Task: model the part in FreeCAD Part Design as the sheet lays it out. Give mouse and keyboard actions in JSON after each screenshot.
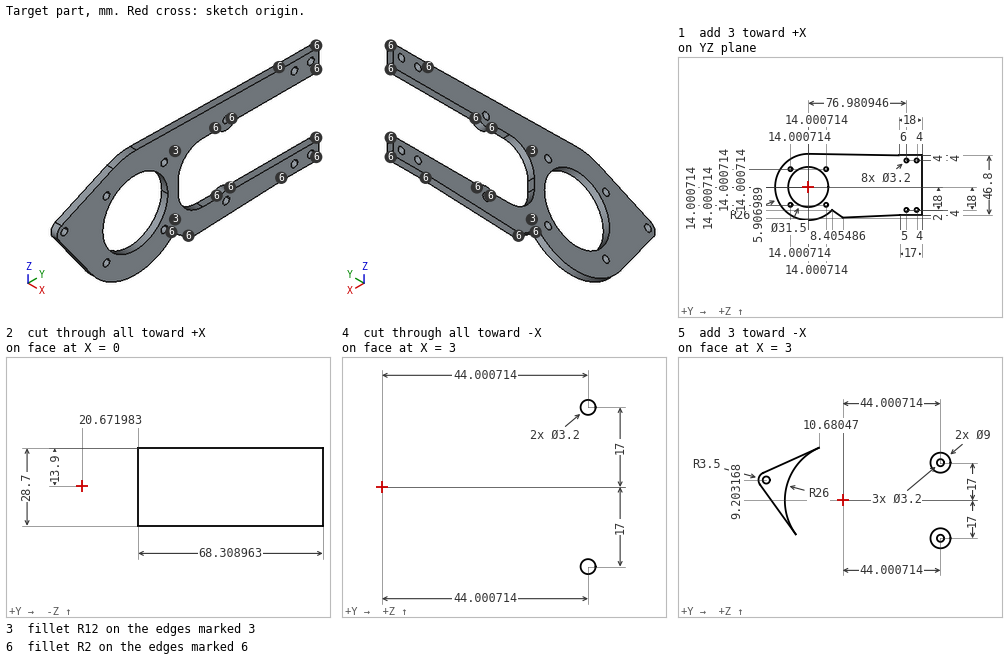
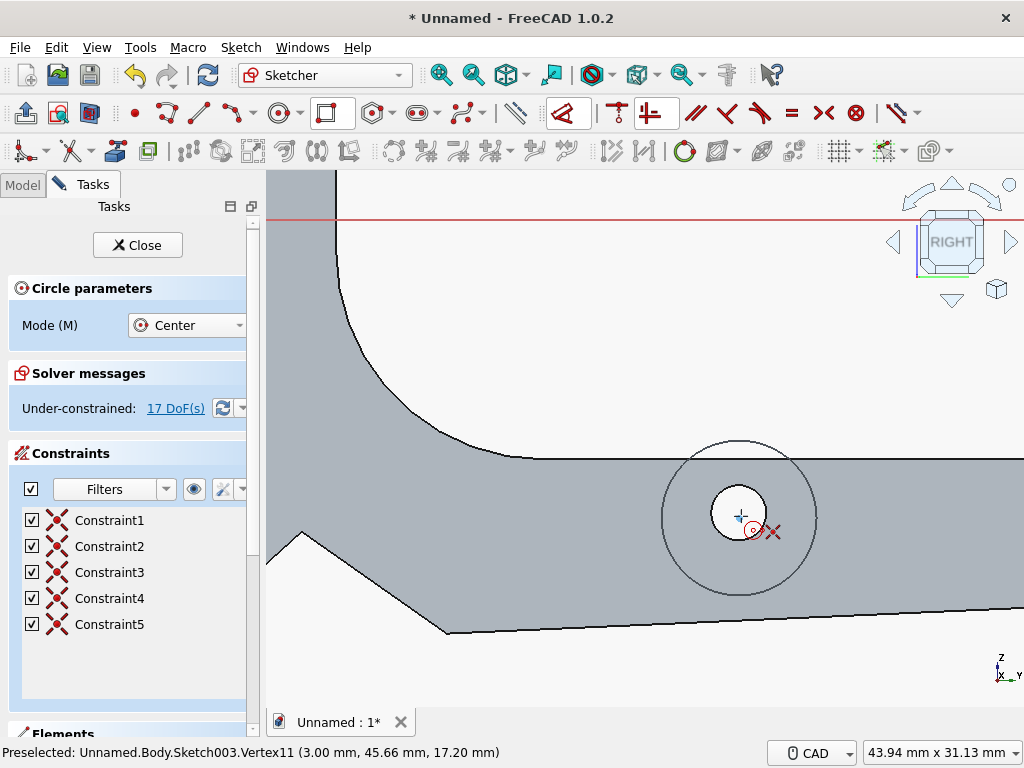
{"action": "scroll", "coordinate": [741, 516], "scroll_direction": "down", "scroll_amount": 7}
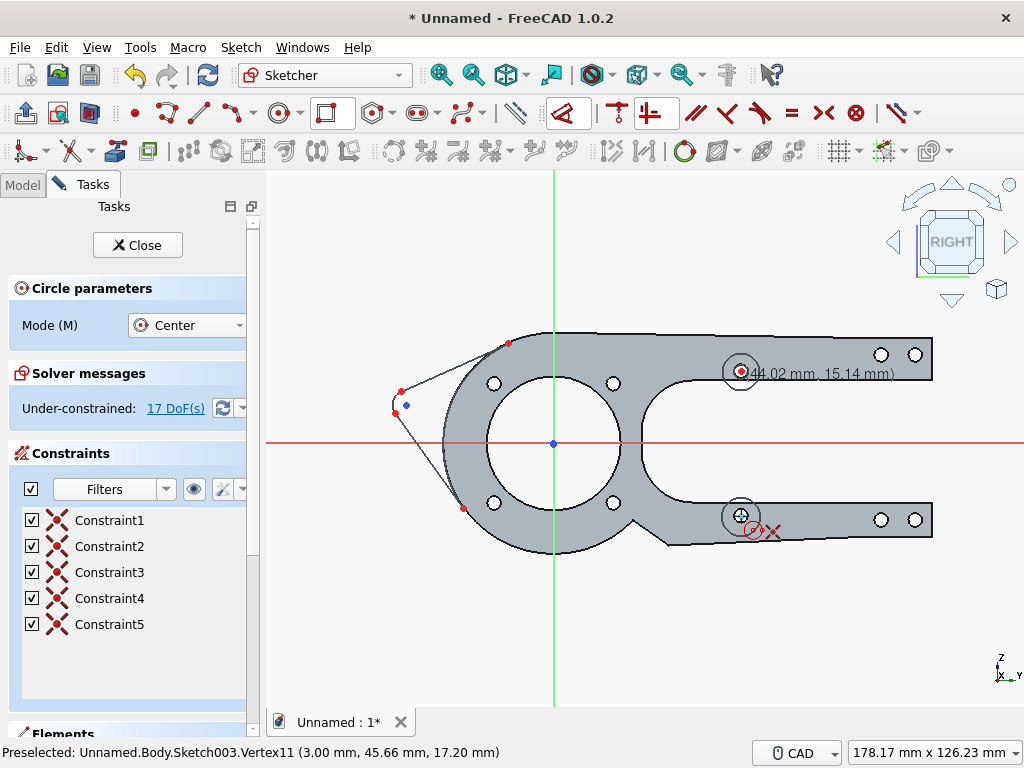
{"action": "left_click", "coordinate": [741, 517]}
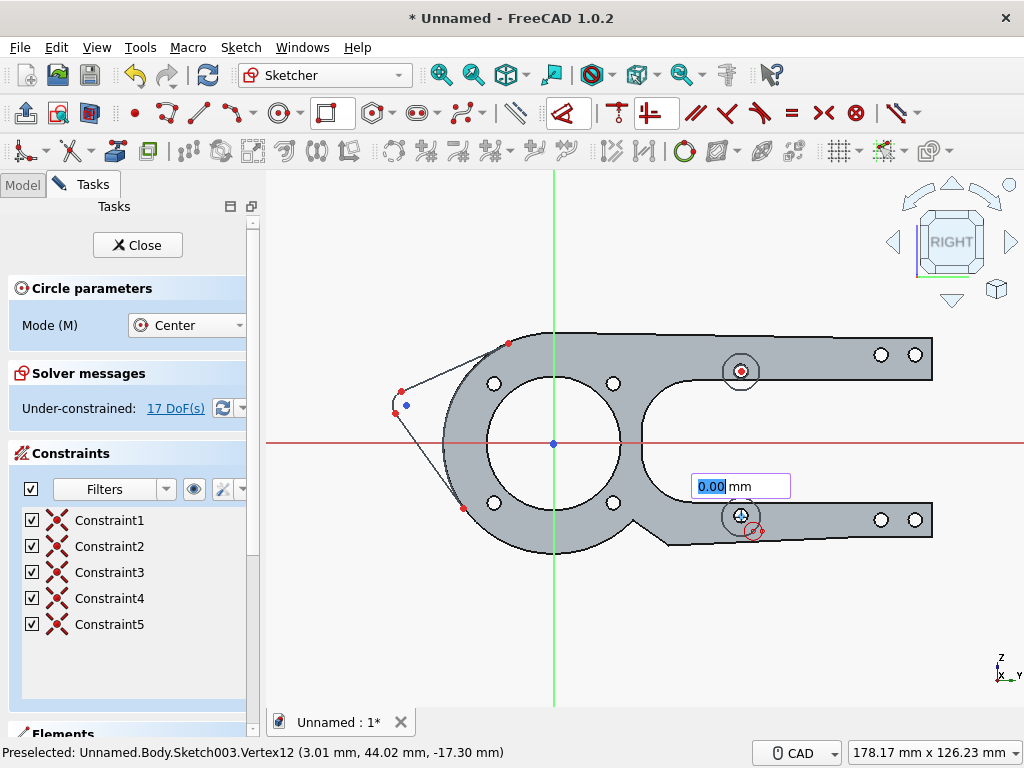
{"action": "scroll", "coordinate": [747, 513], "scroll_direction": "up", "scroll_amount": 5}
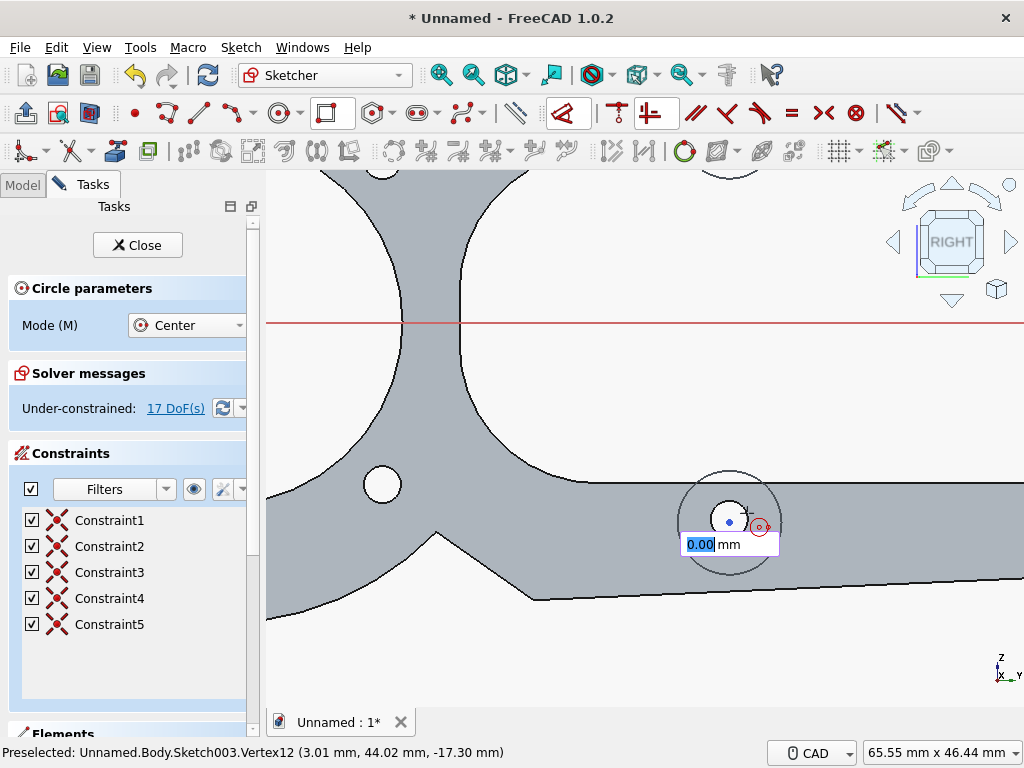
{"action": "left_click", "coordinate": [747, 513]}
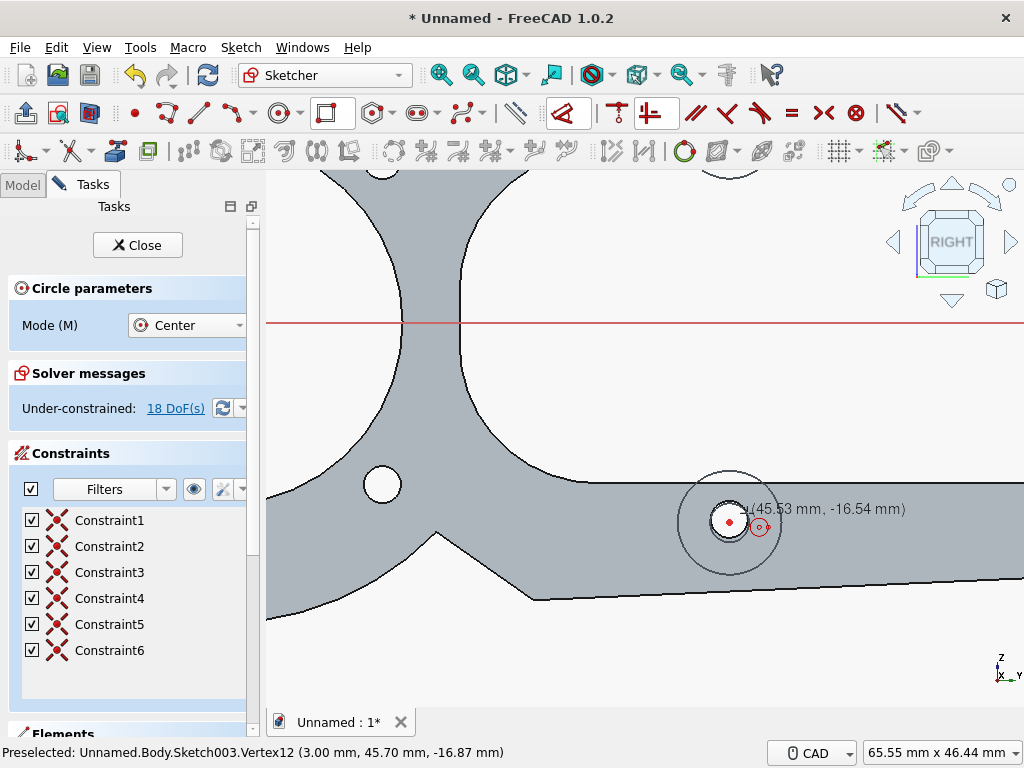
{"action": "scroll", "coordinate": [747, 513], "scroll_direction": "down", "scroll_amount": 5}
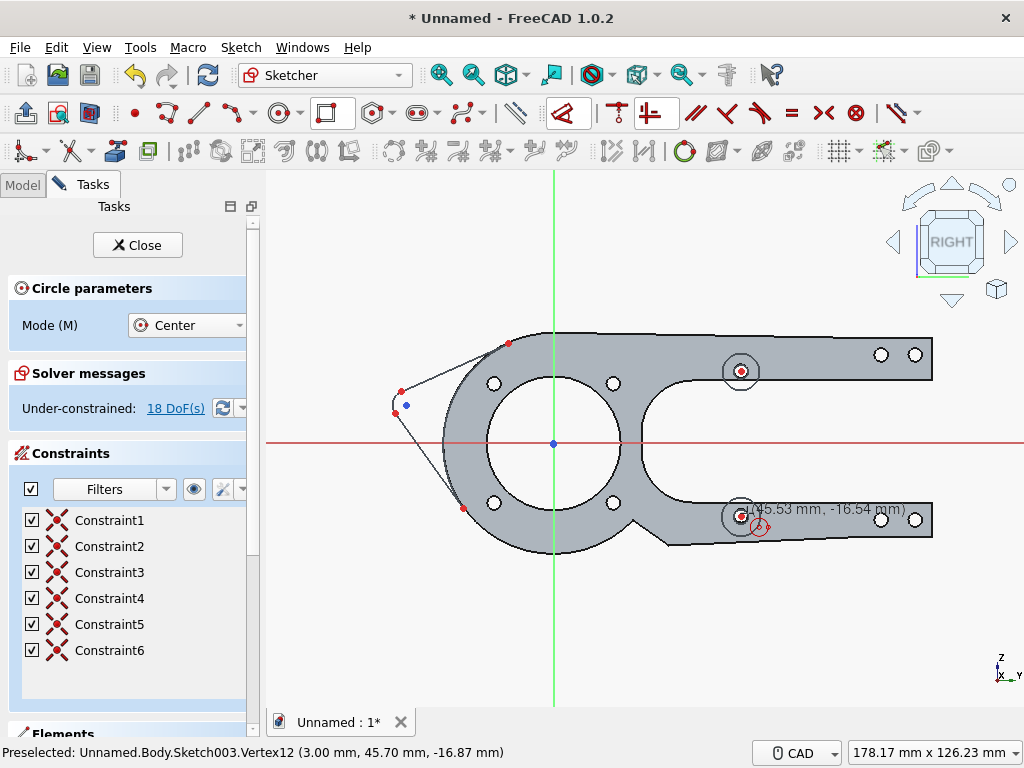
{"action": "scroll", "coordinate": [408, 404], "scroll_direction": "up", "scroll_amount": 7}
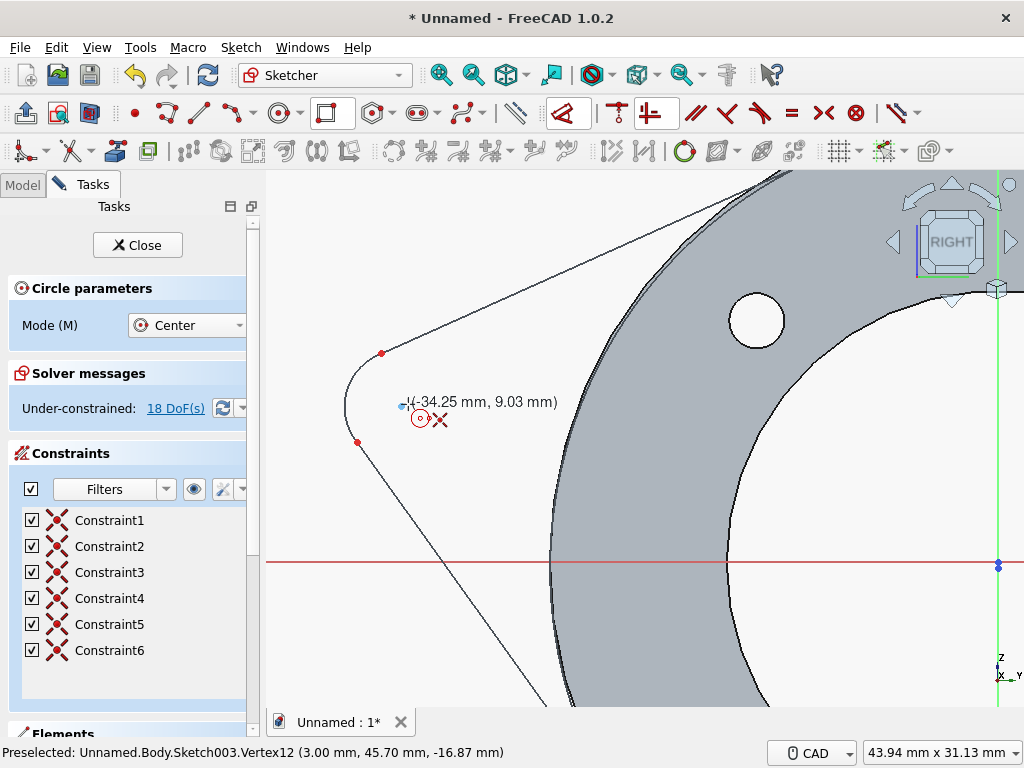
{"action": "scroll", "coordinate": [408, 404], "scroll_direction": "down", "scroll_amount": 7}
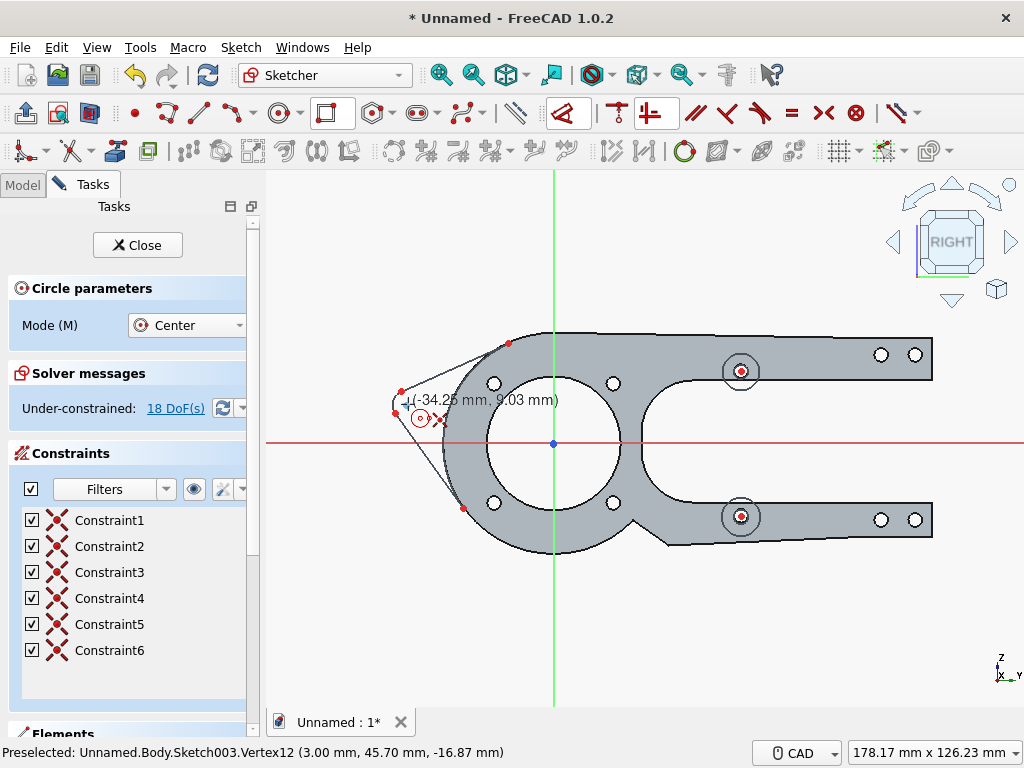
{"action": "left_click", "coordinate": [408, 404]}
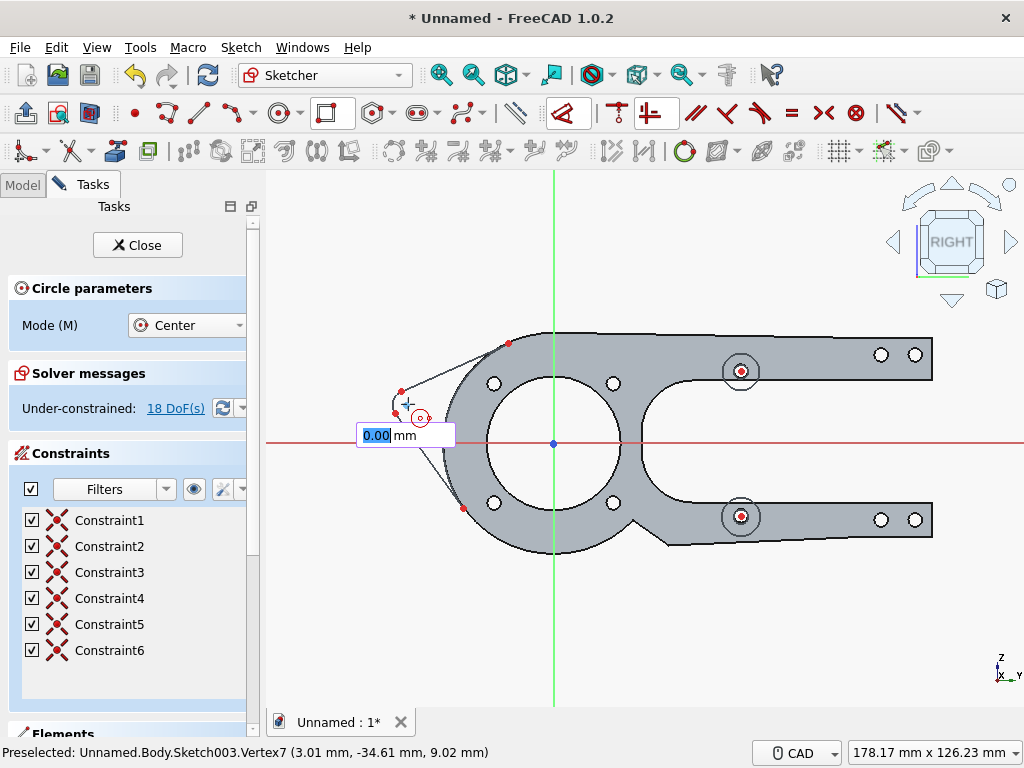
{"action": "scroll", "coordinate": [405, 411], "scroll_direction": "up", "scroll_amount": 5}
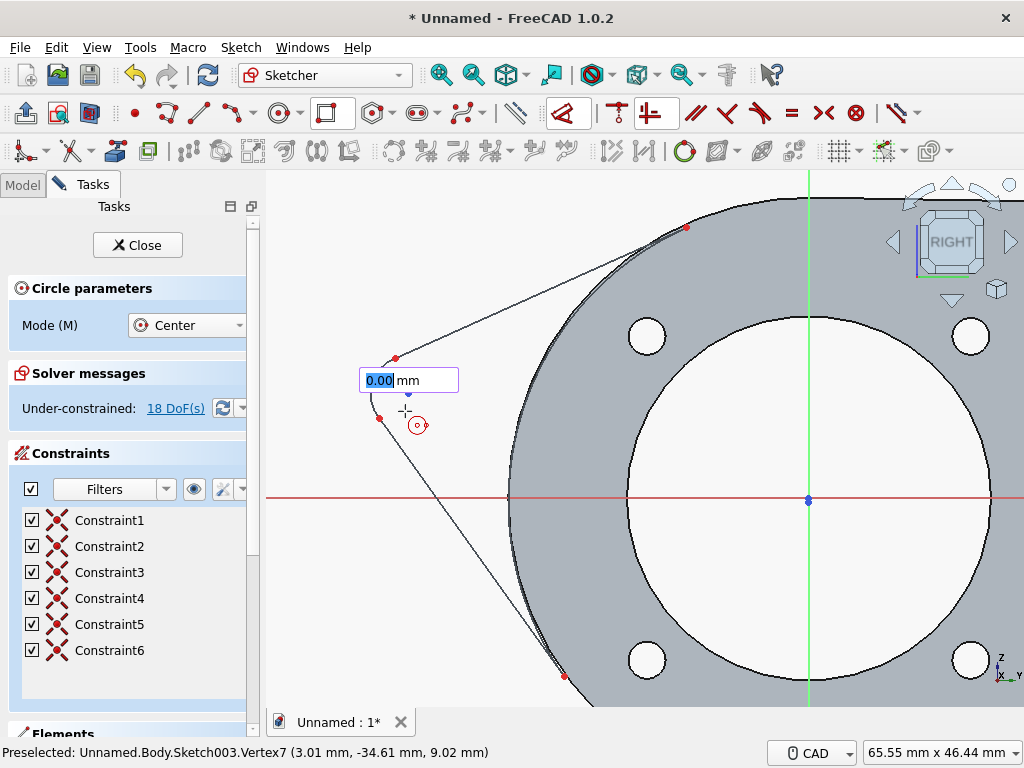
{"action": "left_click", "coordinate": [405, 409]}
{"action": "key", "text": "Escape"}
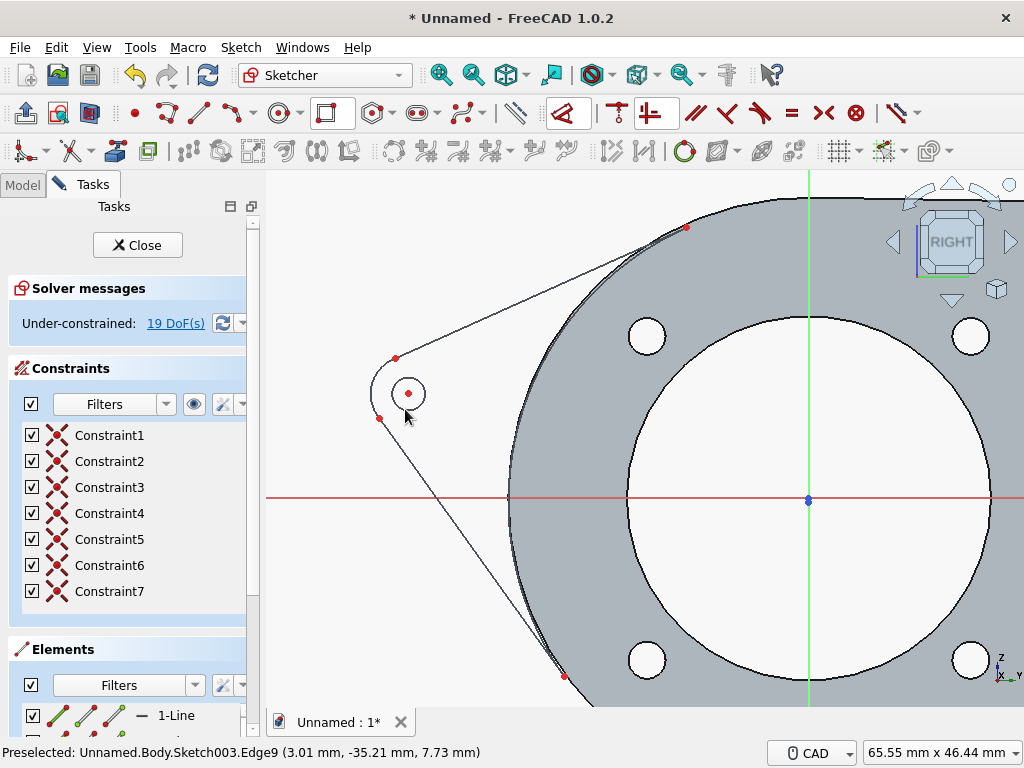
{"action": "left_click", "coordinate": [599, 267]}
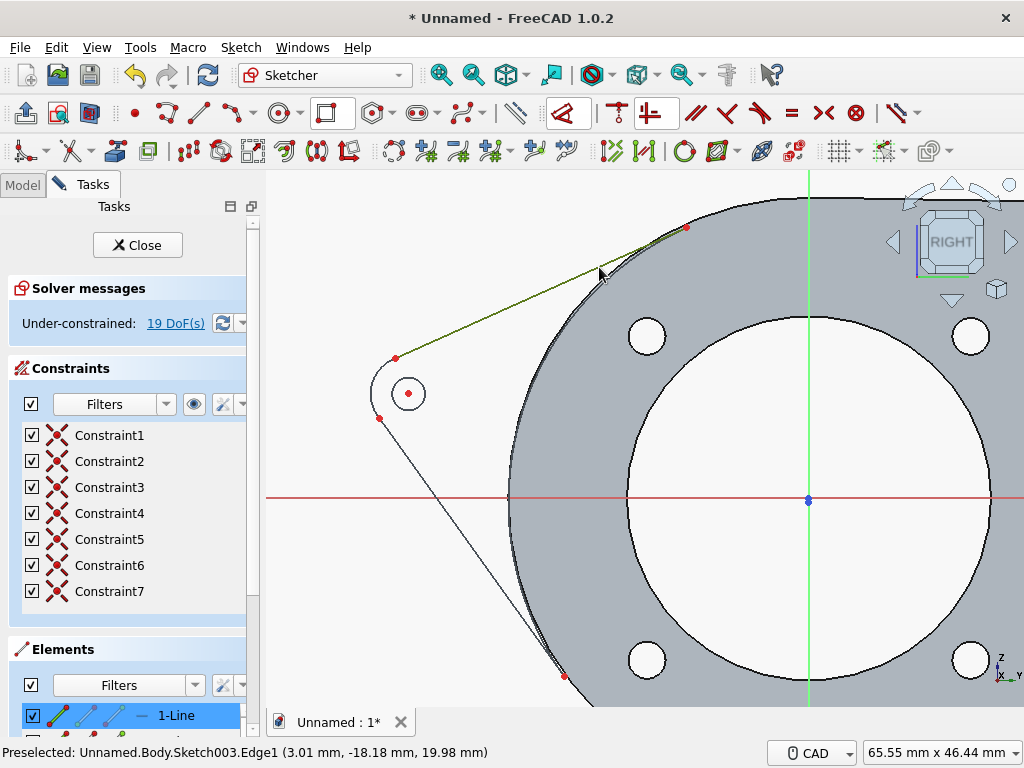
{"action": "left_click", "coordinate": [378, 371]}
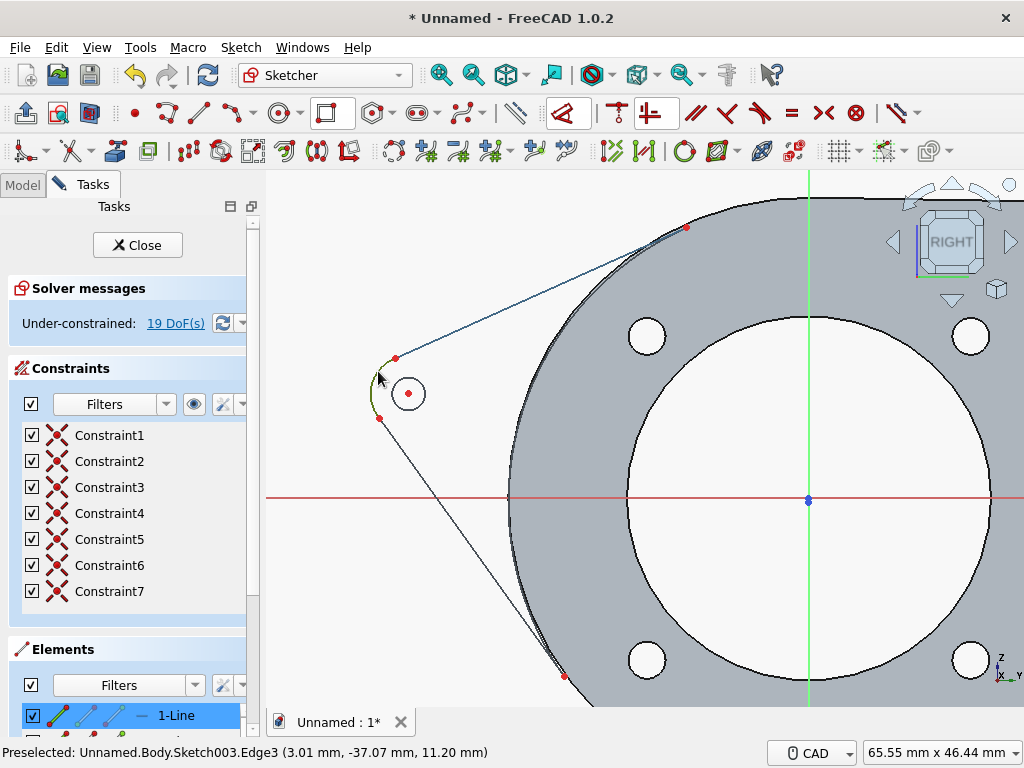
{"action": "left_click", "coordinate": [760, 114]}